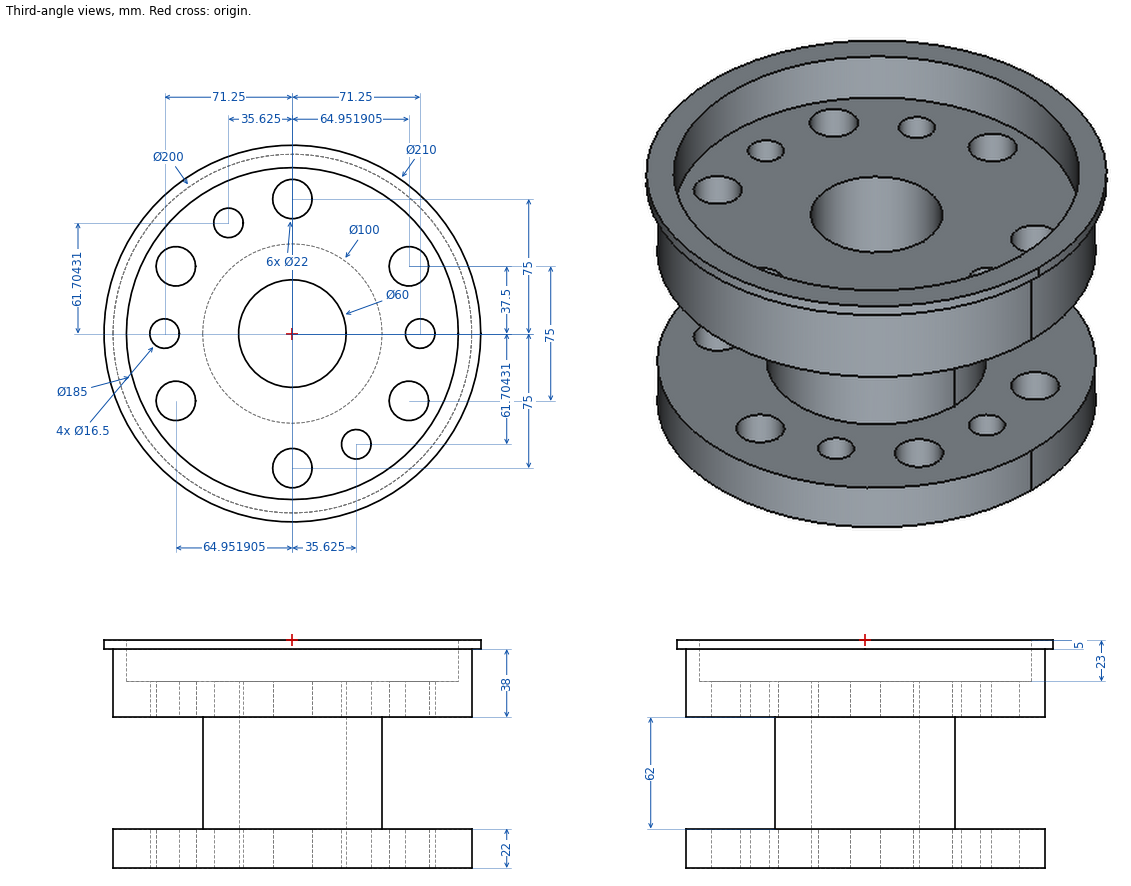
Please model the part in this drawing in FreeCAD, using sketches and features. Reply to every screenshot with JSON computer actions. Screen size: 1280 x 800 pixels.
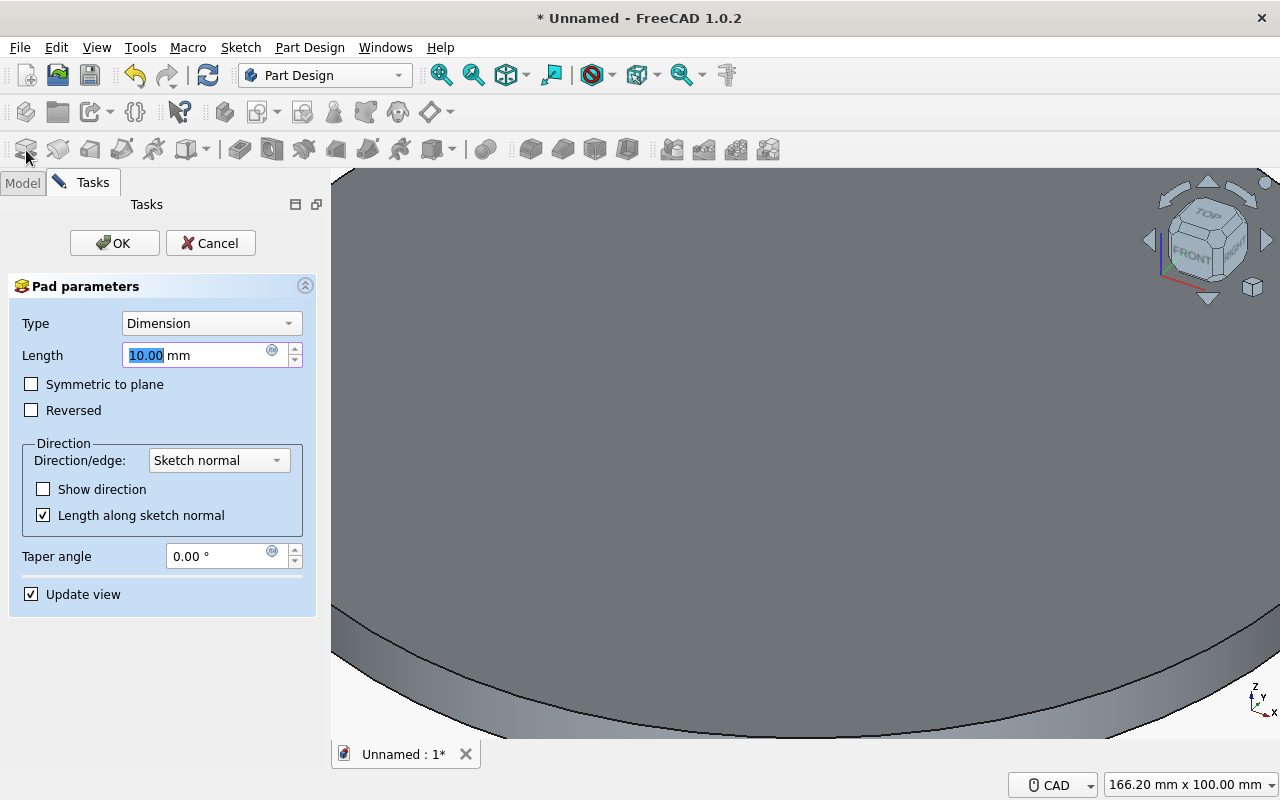
{"action": "type", "text": "5"}
{"action": "key", "text": "Tab"}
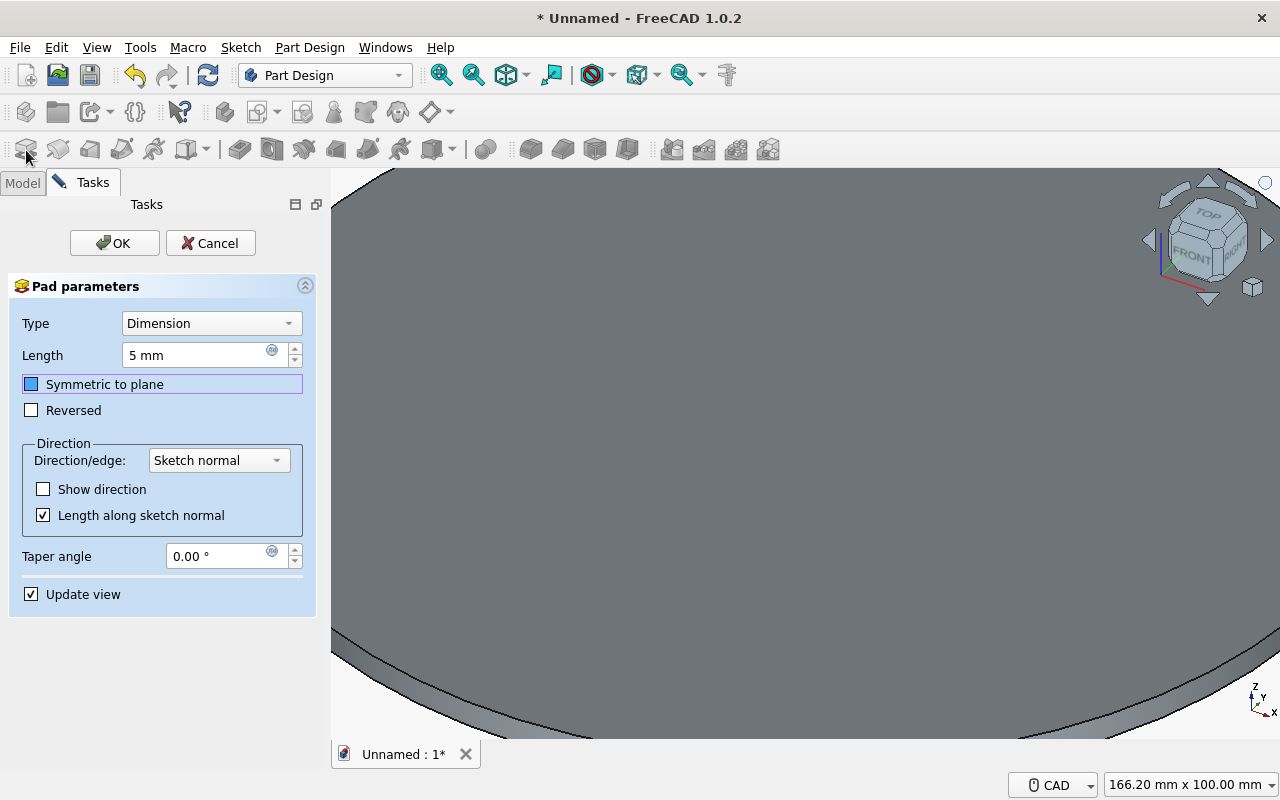
{"action": "left_click", "coordinate": [30, 410]}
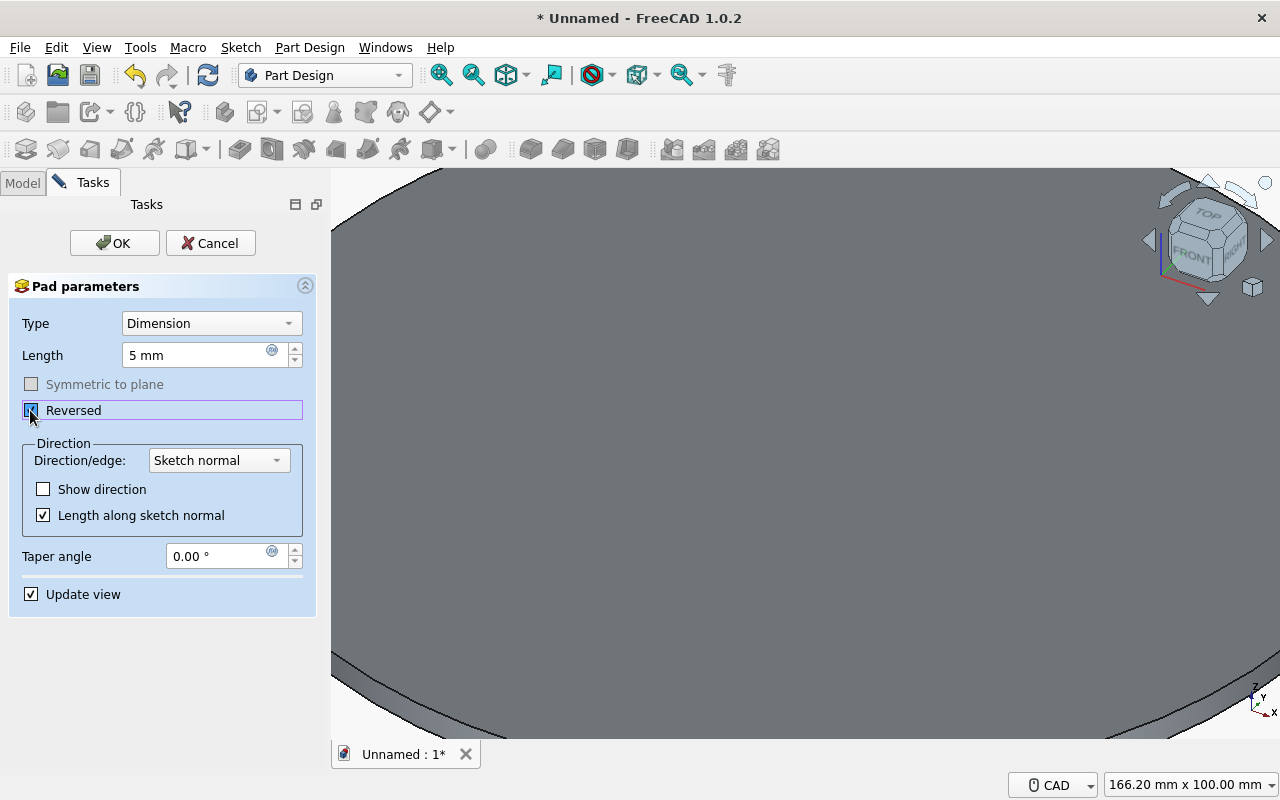
{"action": "left_click", "coordinate": [115, 243]}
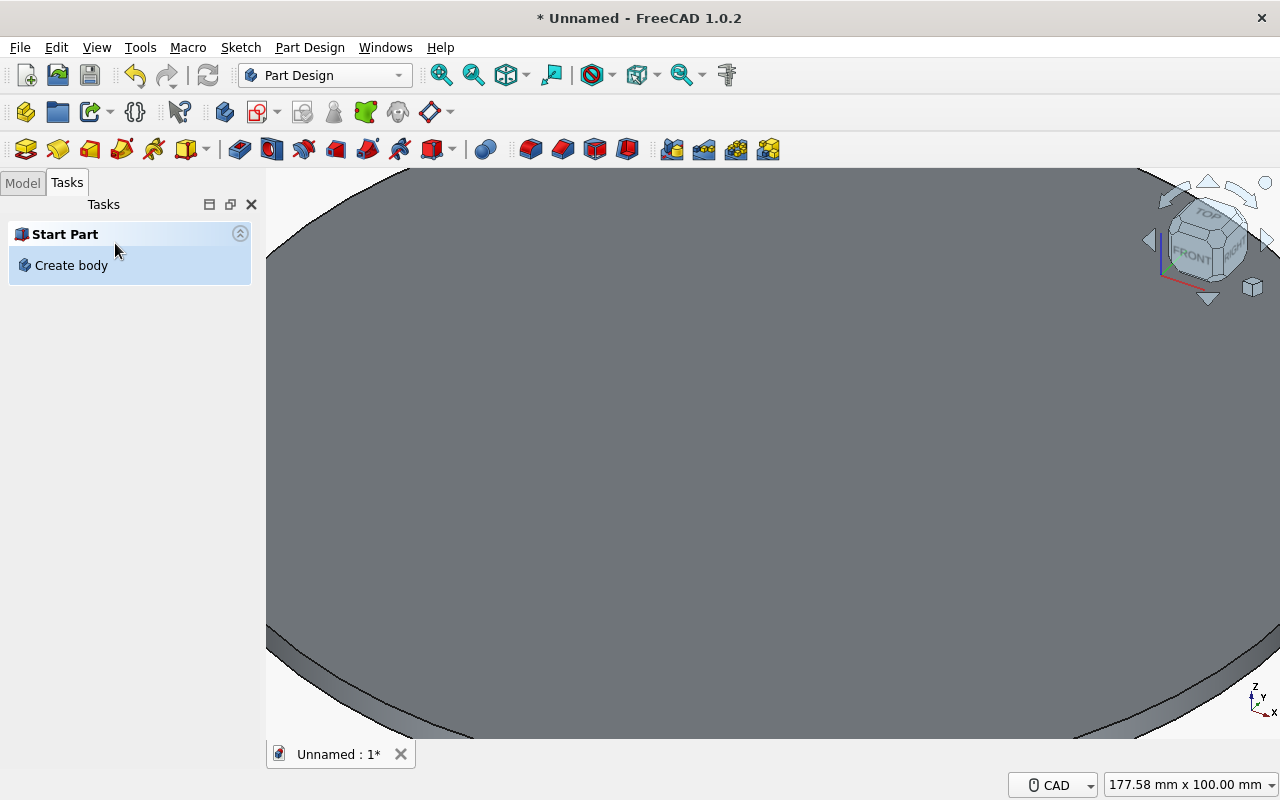
{"action": "left_click", "coordinate": [442, 76]}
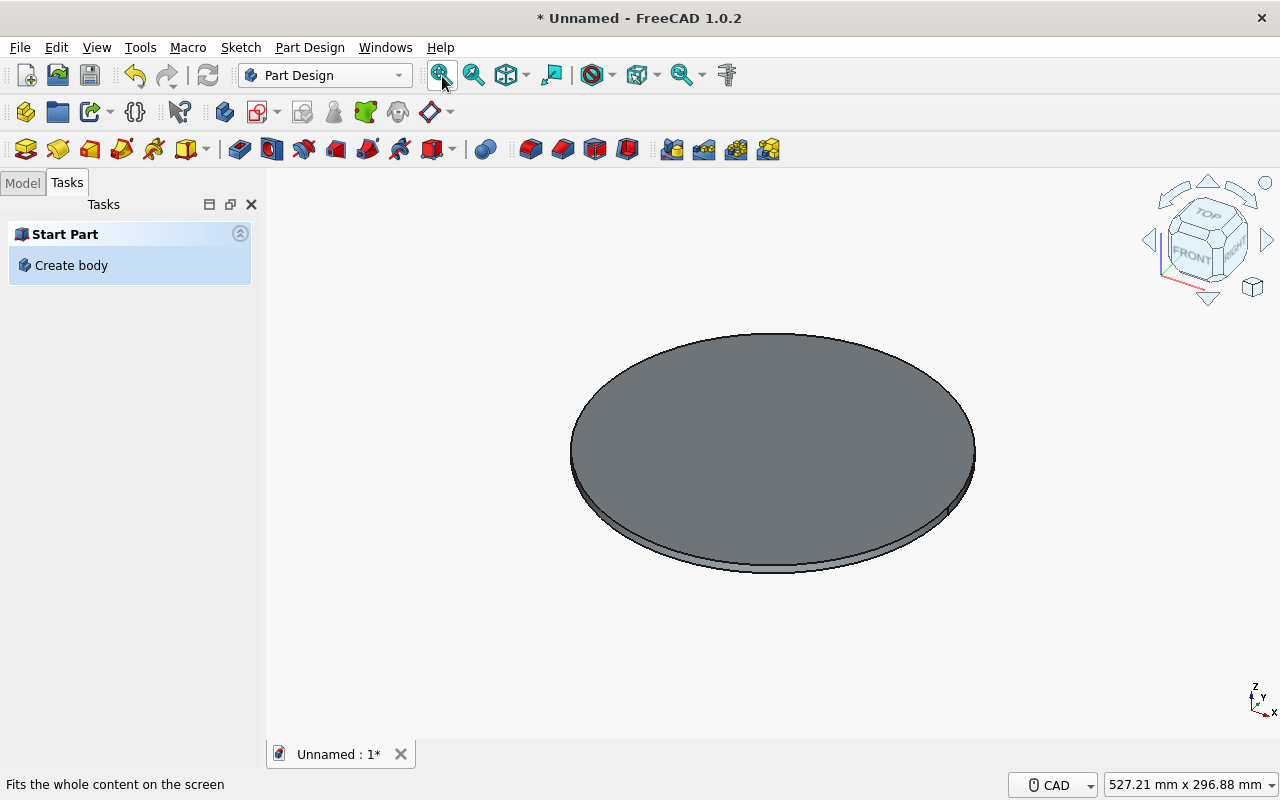
{"action": "key", "text": "5"}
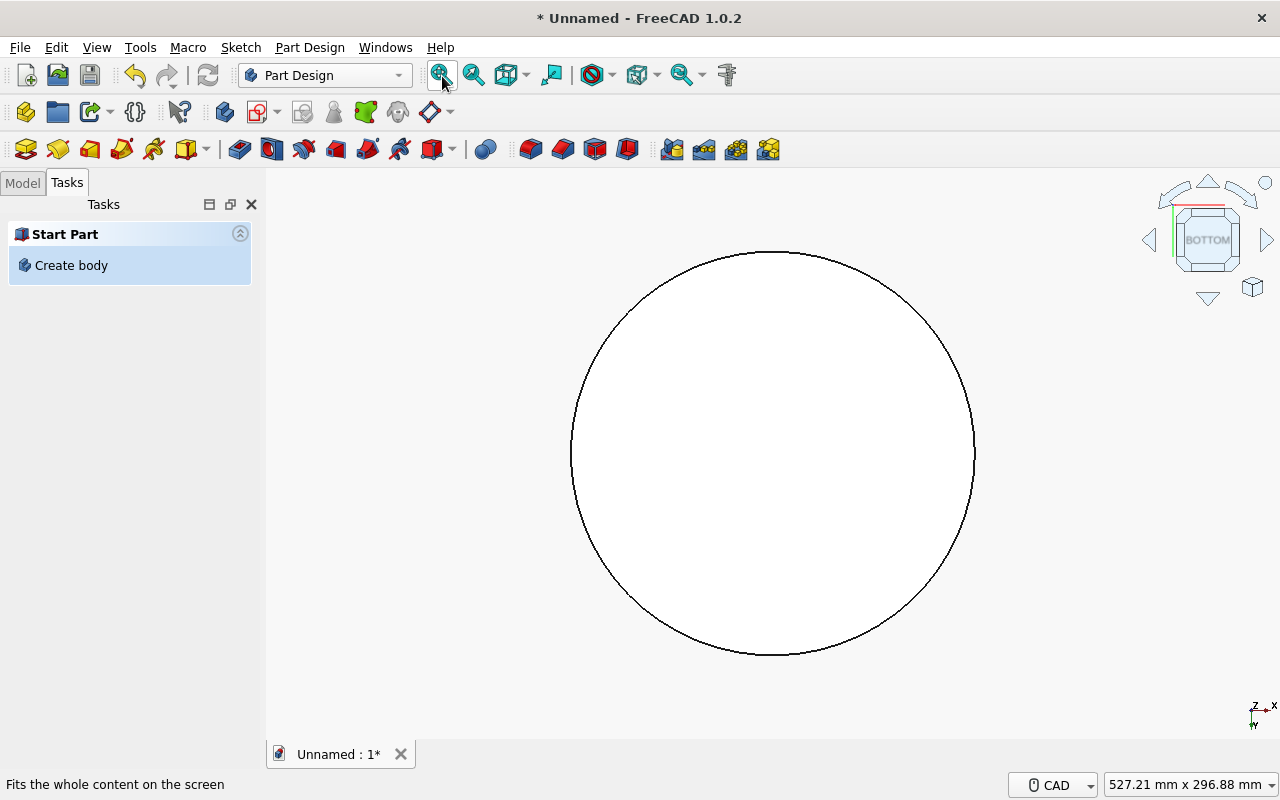
{"action": "left_click", "coordinate": [773, 452]}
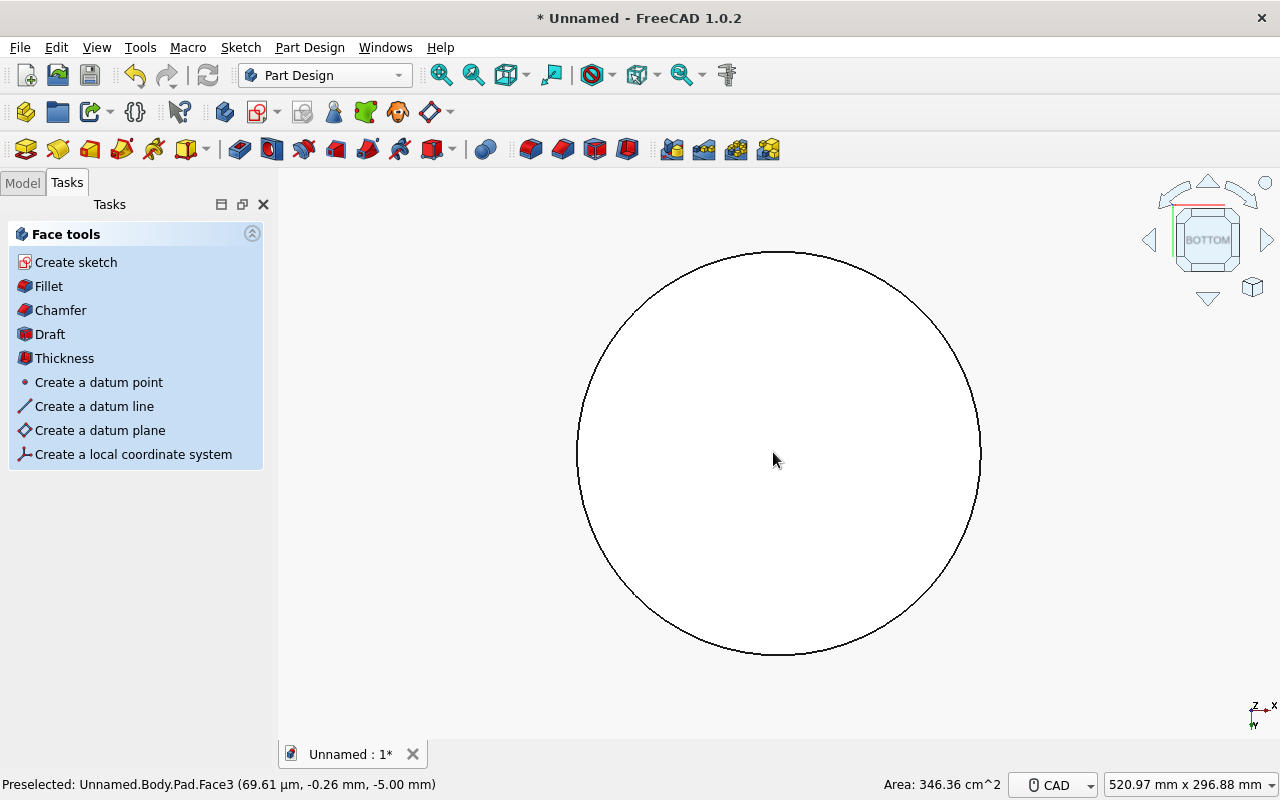
{"action": "left_click", "coordinate": [258, 112]}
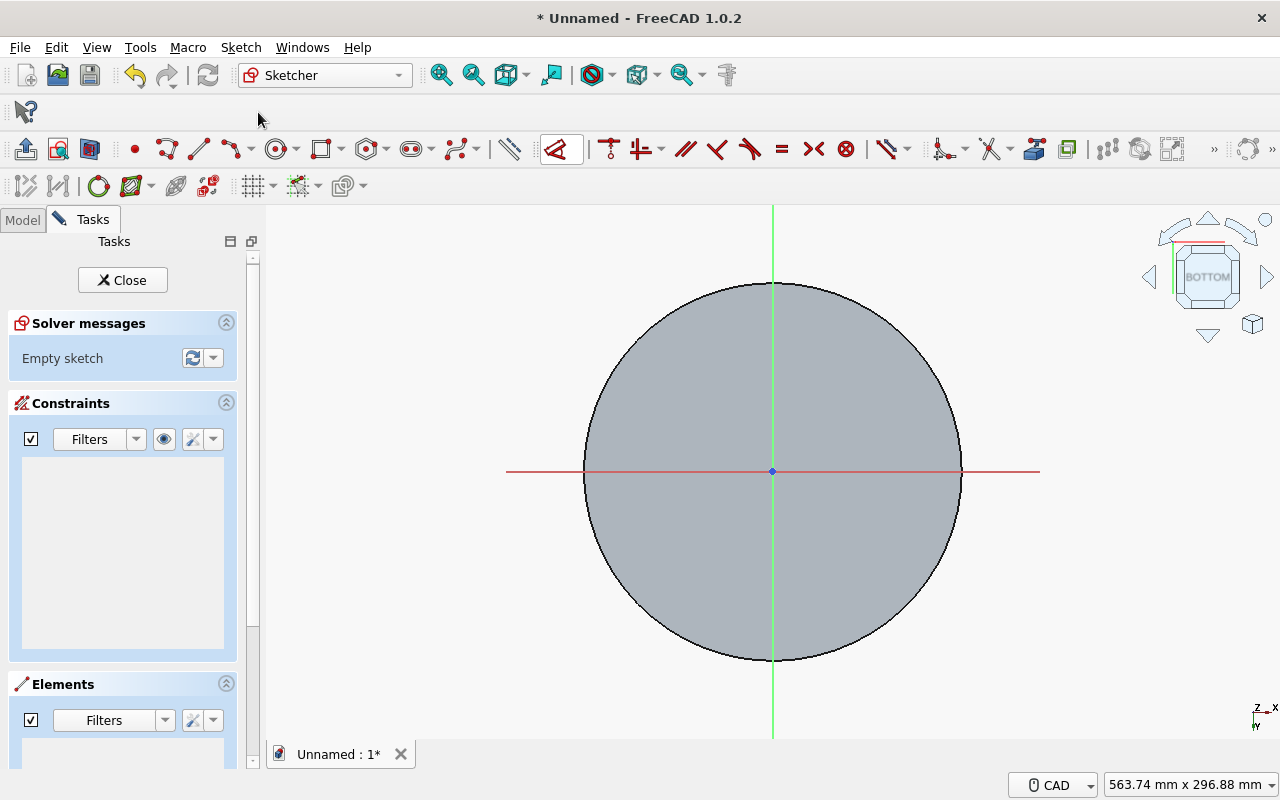
{"action": "left_click", "coordinate": [276, 150]}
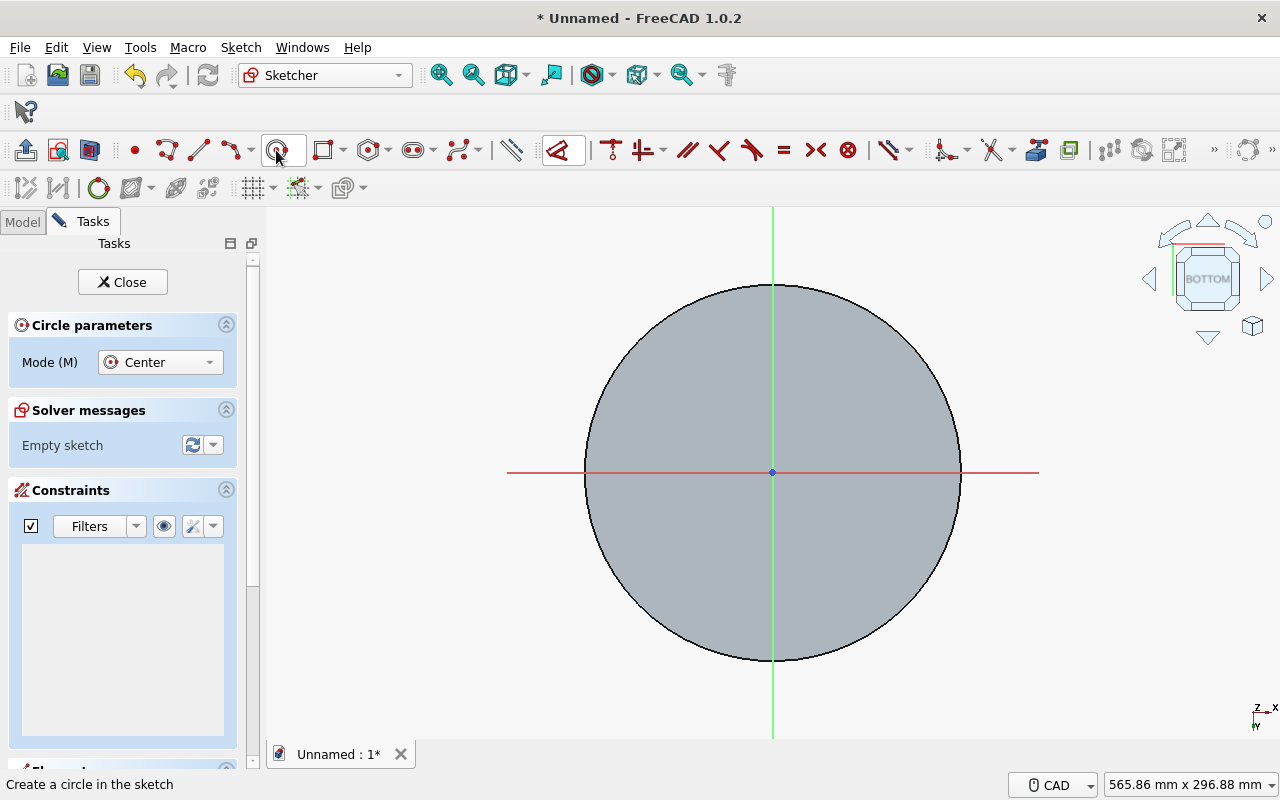
{"action": "left_click", "coordinate": [773, 473]}
{"action": "mouse_move", "coordinate": [900, 346]}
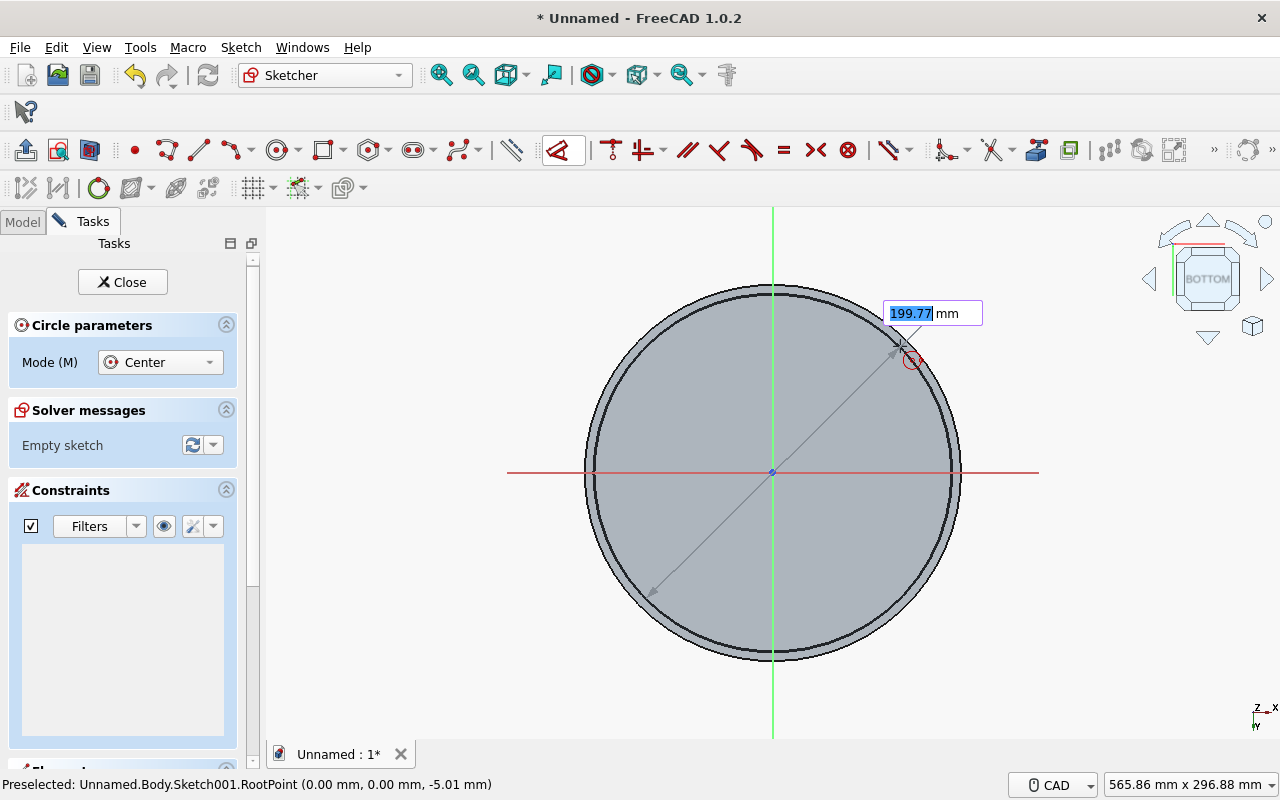
{"action": "type", "text": "200"}
{"action": "key", "text": "Return"}
{"action": "key", "text": "Escape"}